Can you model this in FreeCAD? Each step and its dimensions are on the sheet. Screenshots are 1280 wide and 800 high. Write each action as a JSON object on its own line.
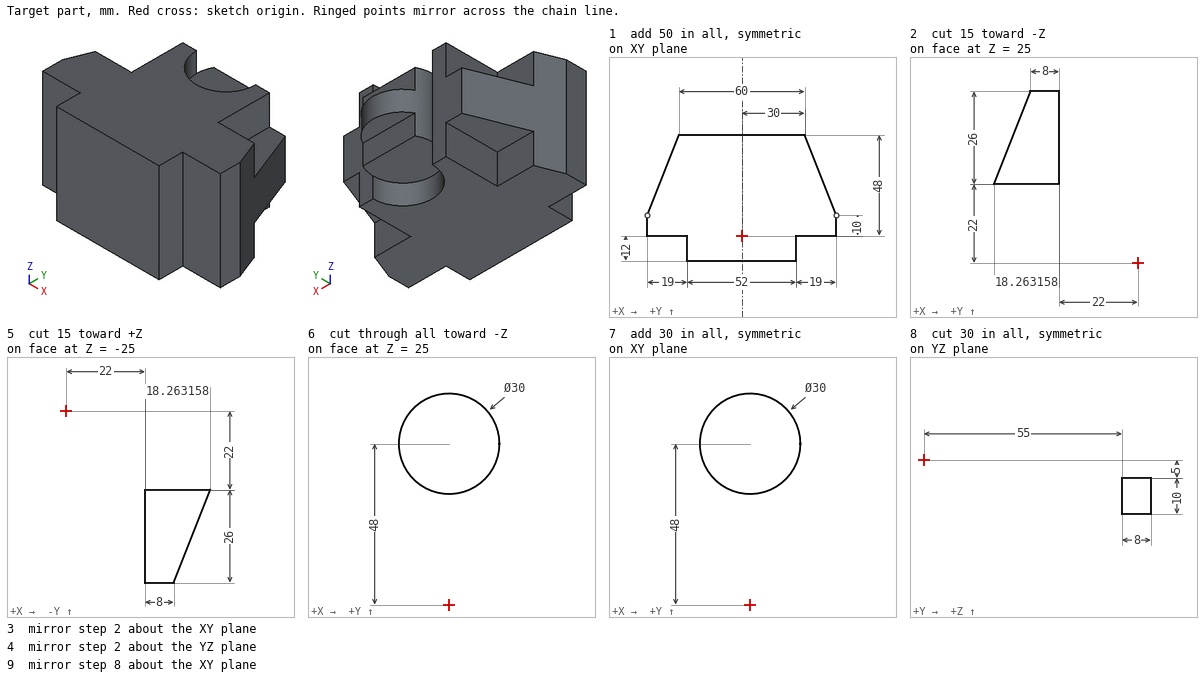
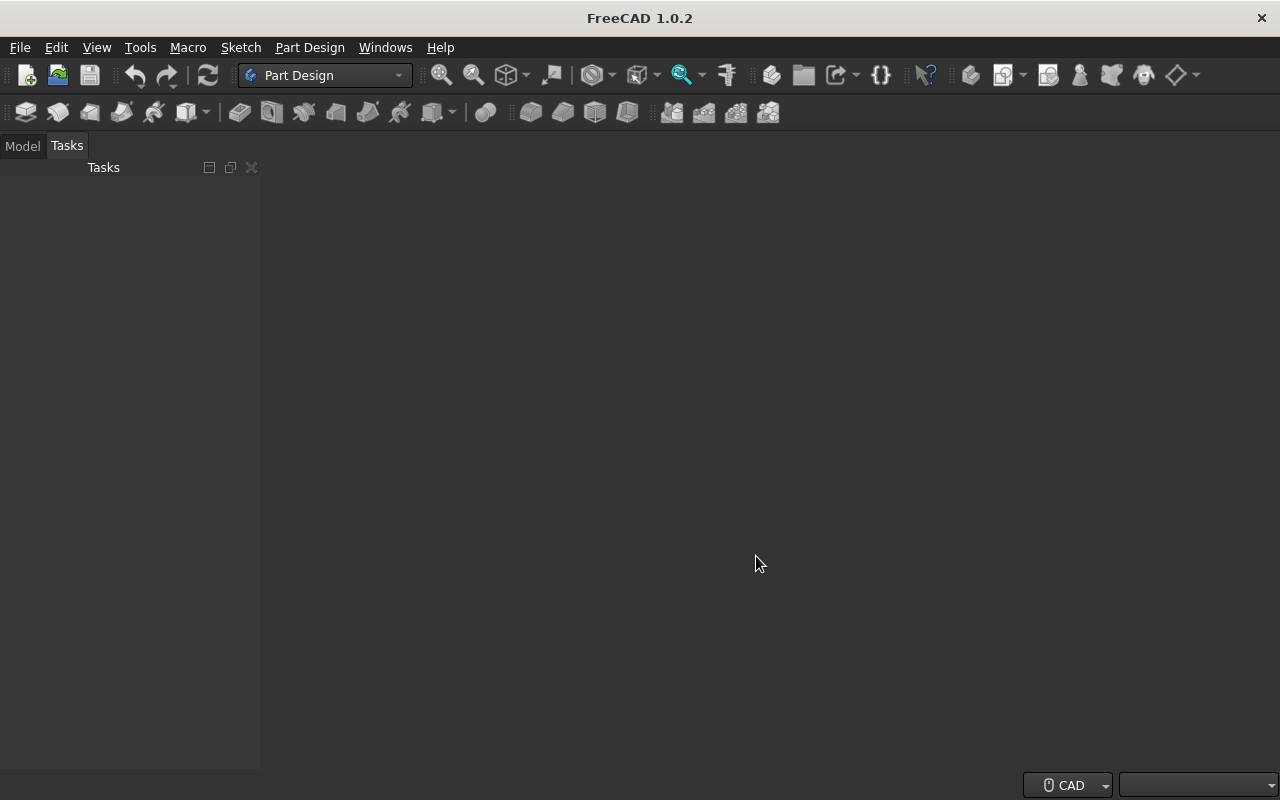
{"action": "key", "text": "ctrl+n"}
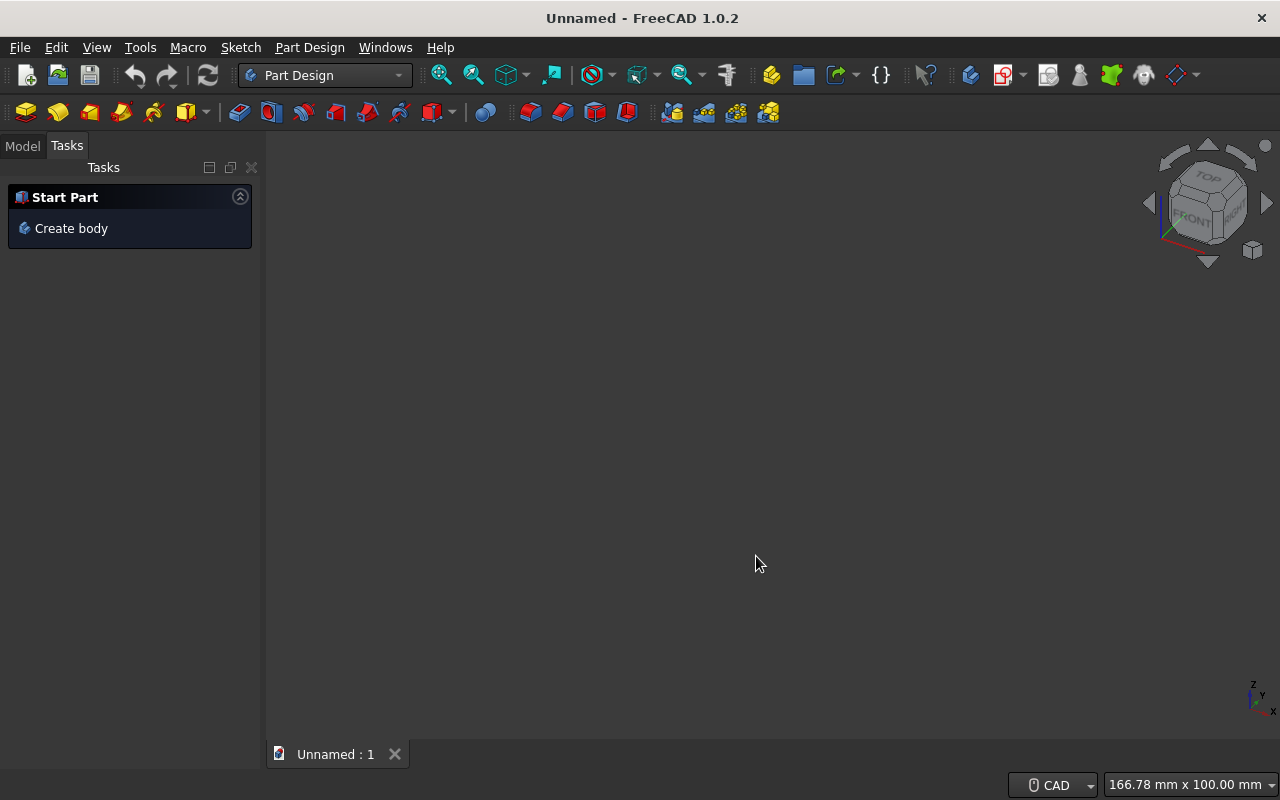
{"action": "left_click", "coordinate": [1004, 76]}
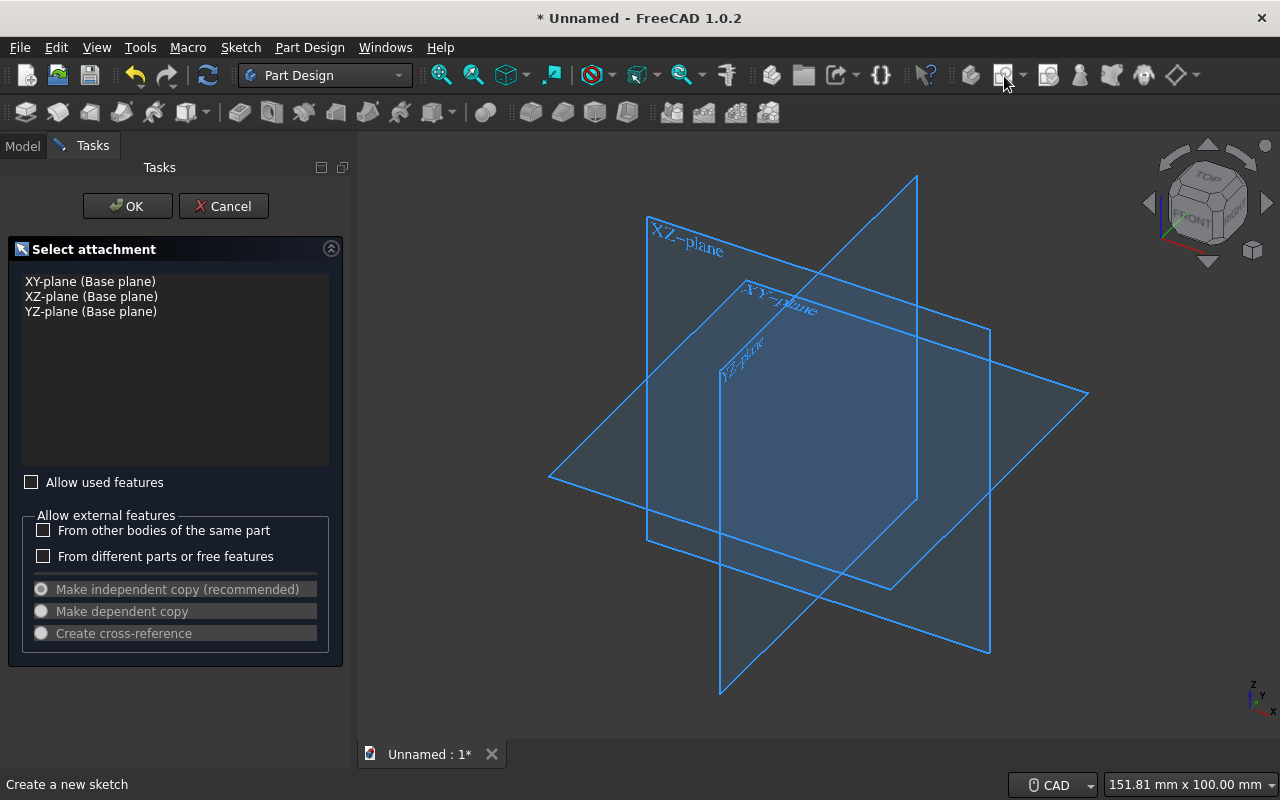
{"action": "left_click", "coordinate": [82, 282]}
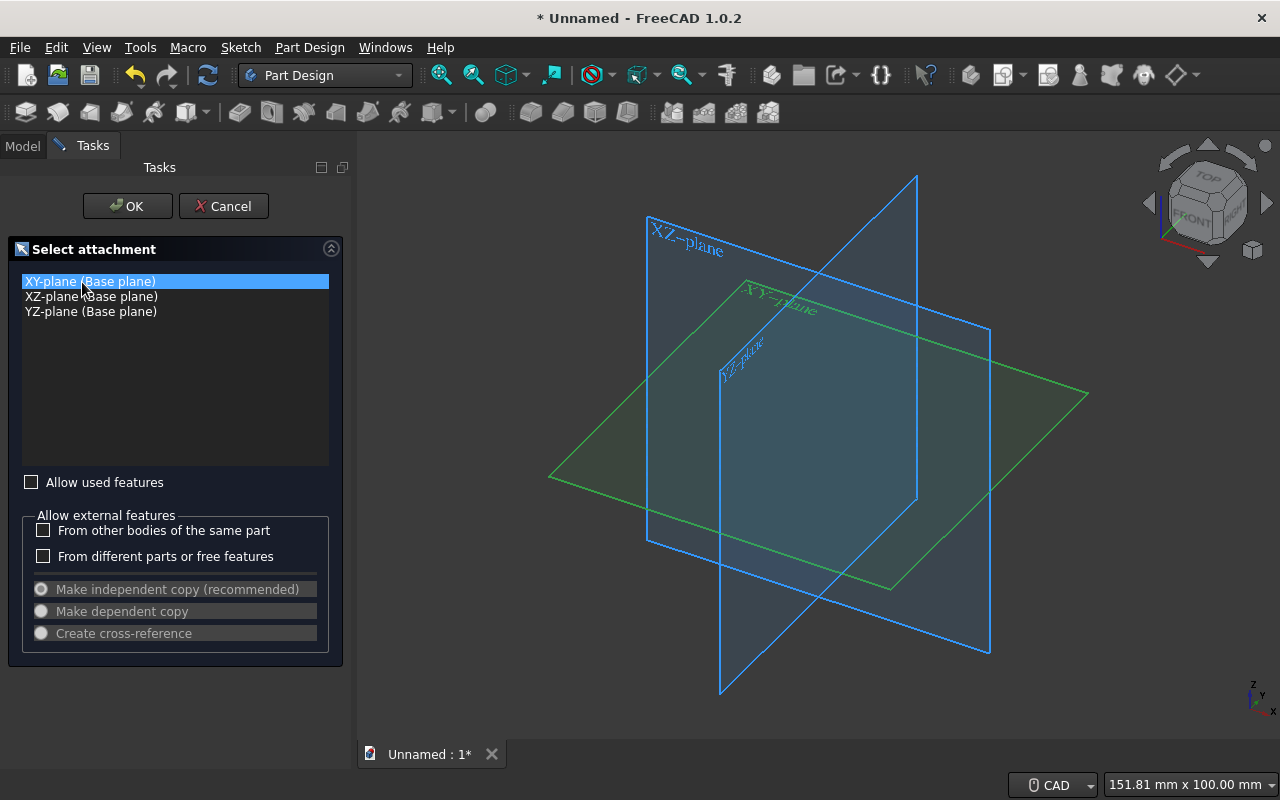
{"action": "left_click", "coordinate": [128, 206]}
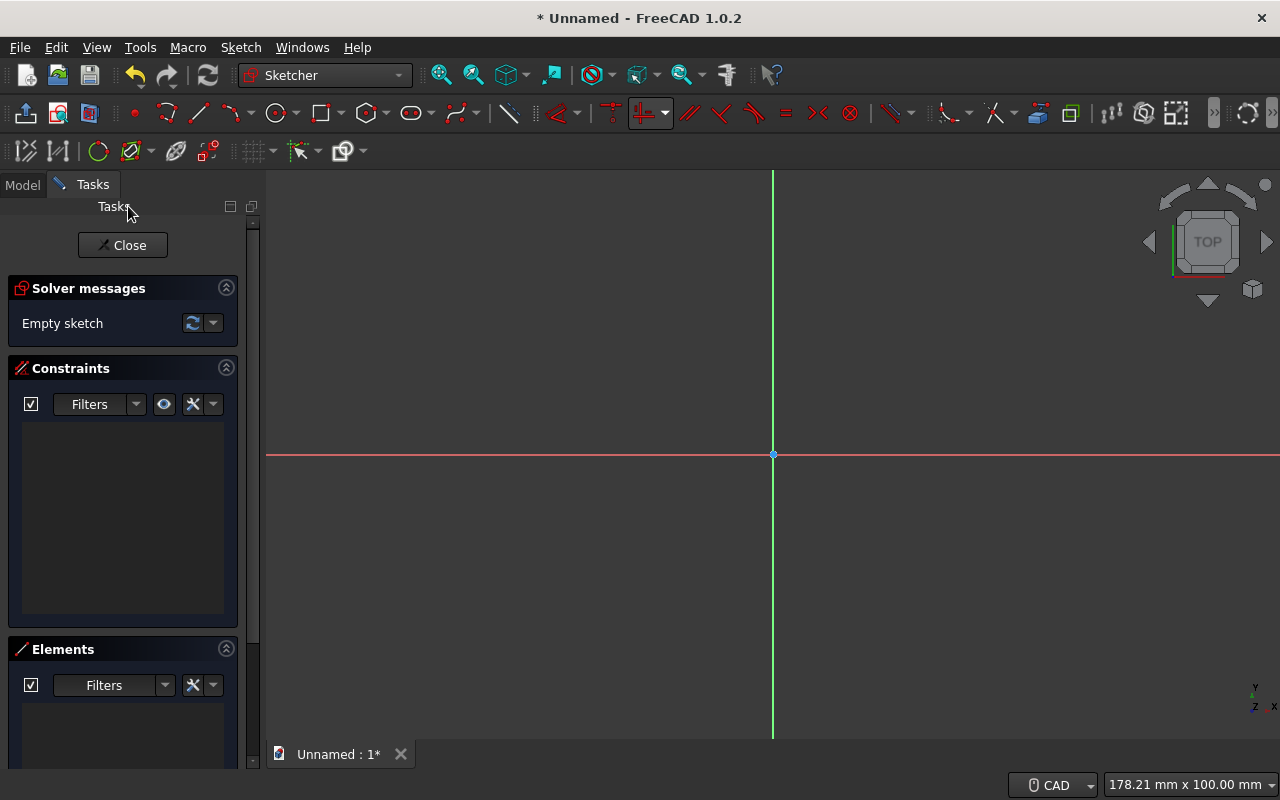
{"action": "scroll", "coordinate": [395, 711], "scroll_direction": "down", "scroll_amount": 1}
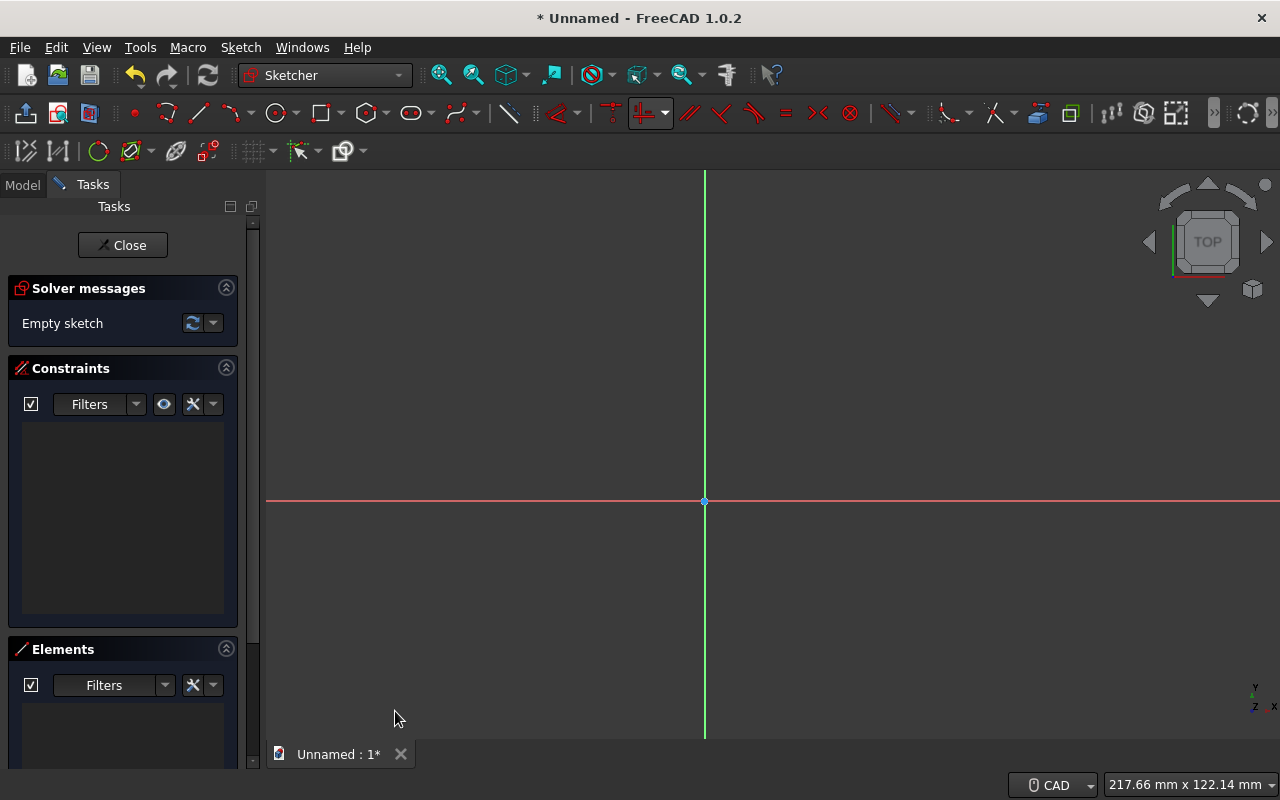
{"action": "left_click", "coordinate": [168, 114]}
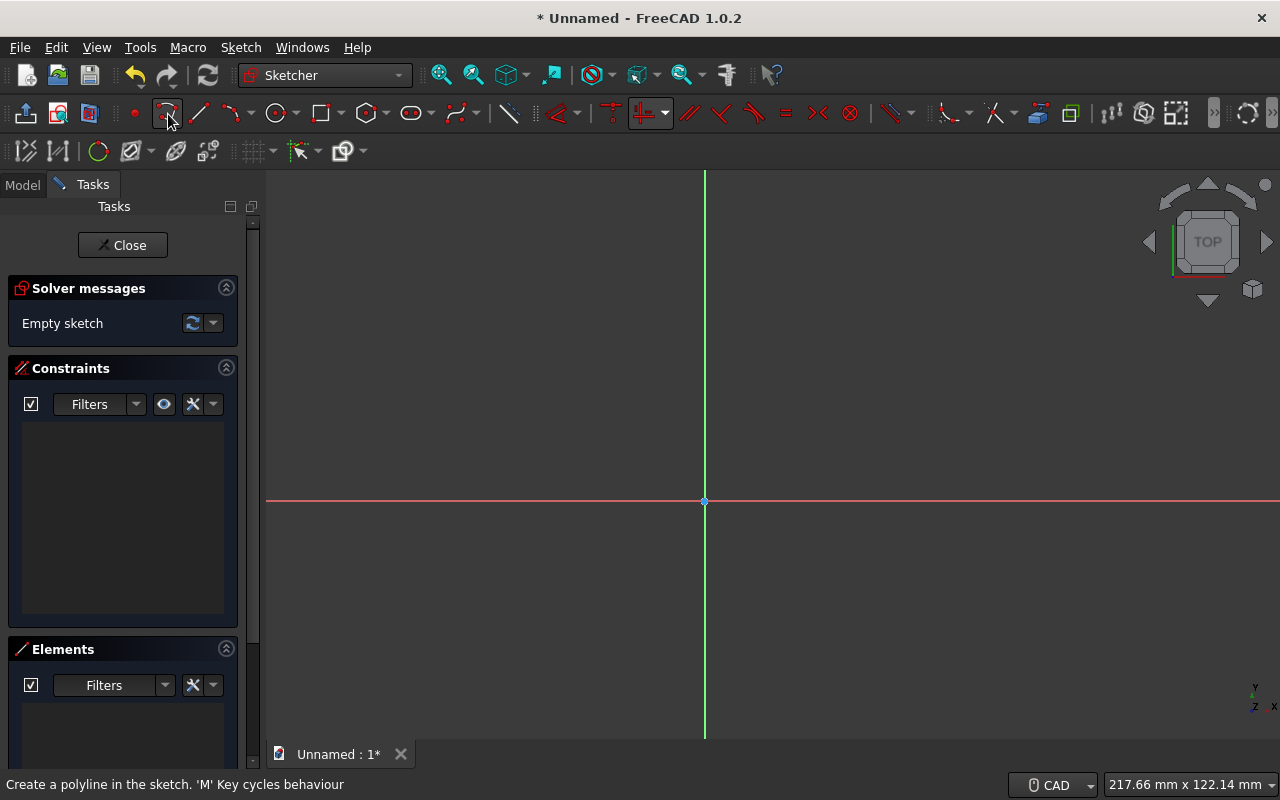
{"action": "left_click", "coordinate": [583, 501]}
{"action": "left_click", "coordinate": [583, 557]}
{"action": "left_click", "coordinate": [826, 557]}
{"action": "left_click", "coordinate": [826, 501]}
{"action": "left_click", "coordinate": [914, 492]}
{"action": "left_click", "coordinate": [914, 455]}
{"action": "left_click", "coordinate": [844, 278]}
{"action": "left_click", "coordinate": [565, 278]}
{"action": "left_click", "coordinate": [495, 455]}
{"action": "left_click", "coordinate": [495, 492]}
{"action": "left_click", "coordinate": [583, 501]}
{"action": "key", "text": "Escape"}
{"action": "key", "text": "Escape"}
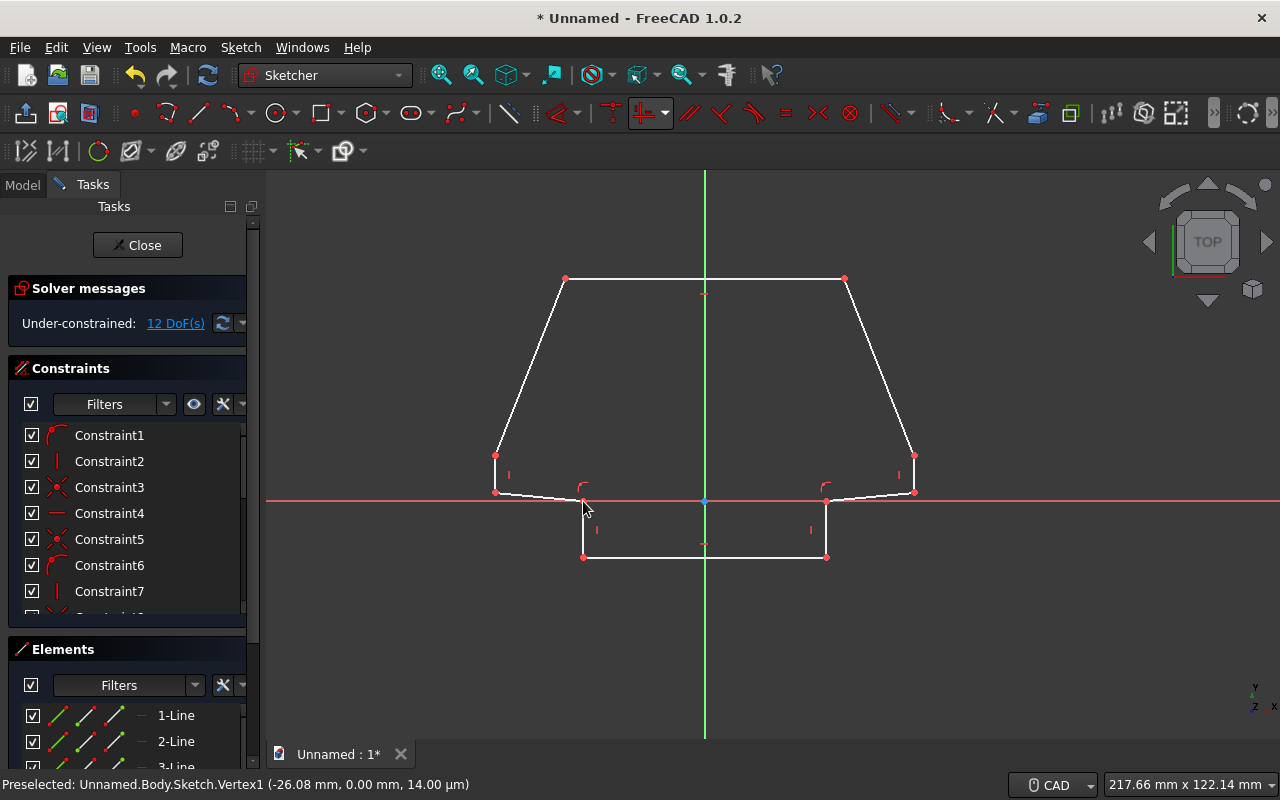
{"action": "left_click", "coordinate": [852, 499]}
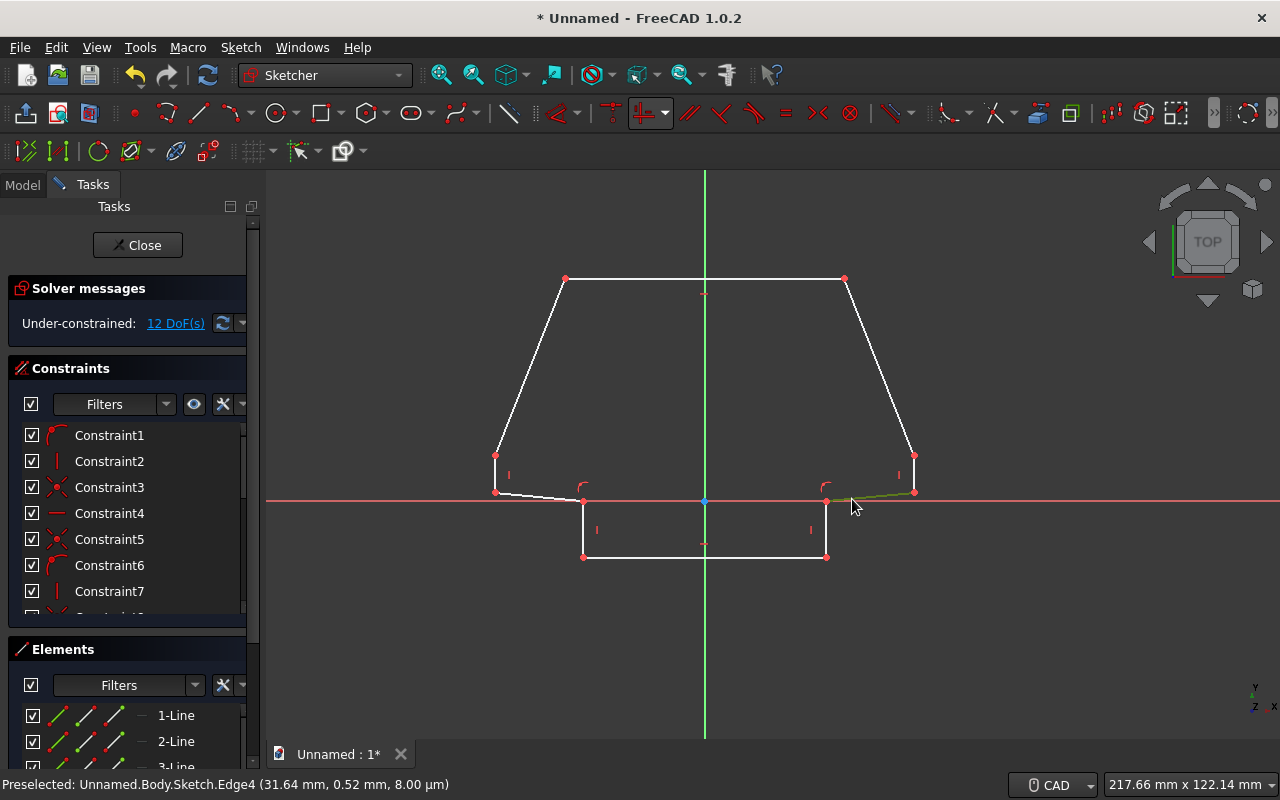
{"action": "key", "text": "h"}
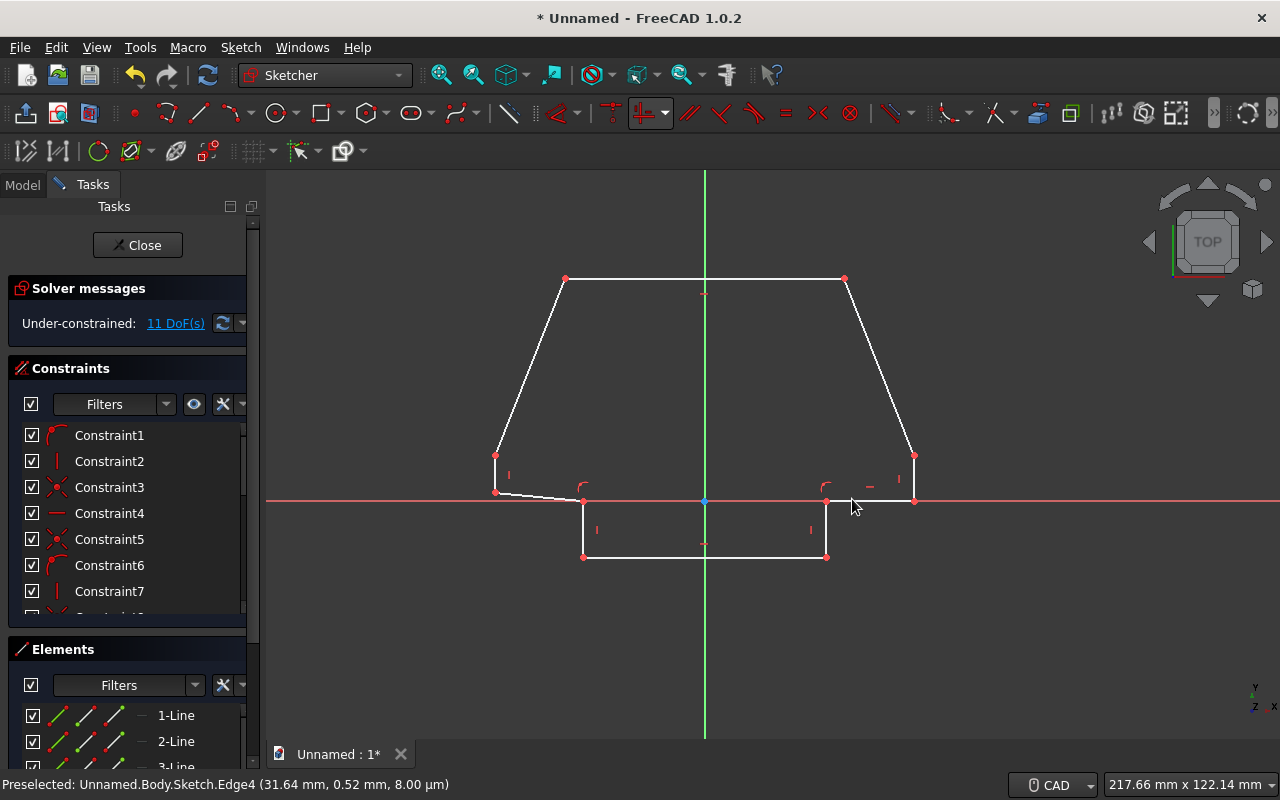
{"action": "left_click", "coordinate": [557, 499]}